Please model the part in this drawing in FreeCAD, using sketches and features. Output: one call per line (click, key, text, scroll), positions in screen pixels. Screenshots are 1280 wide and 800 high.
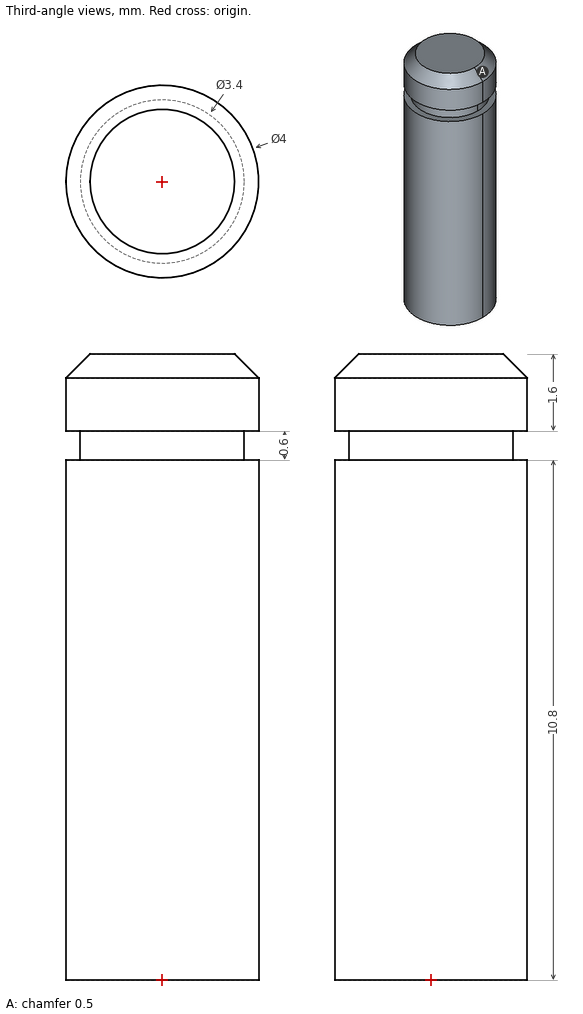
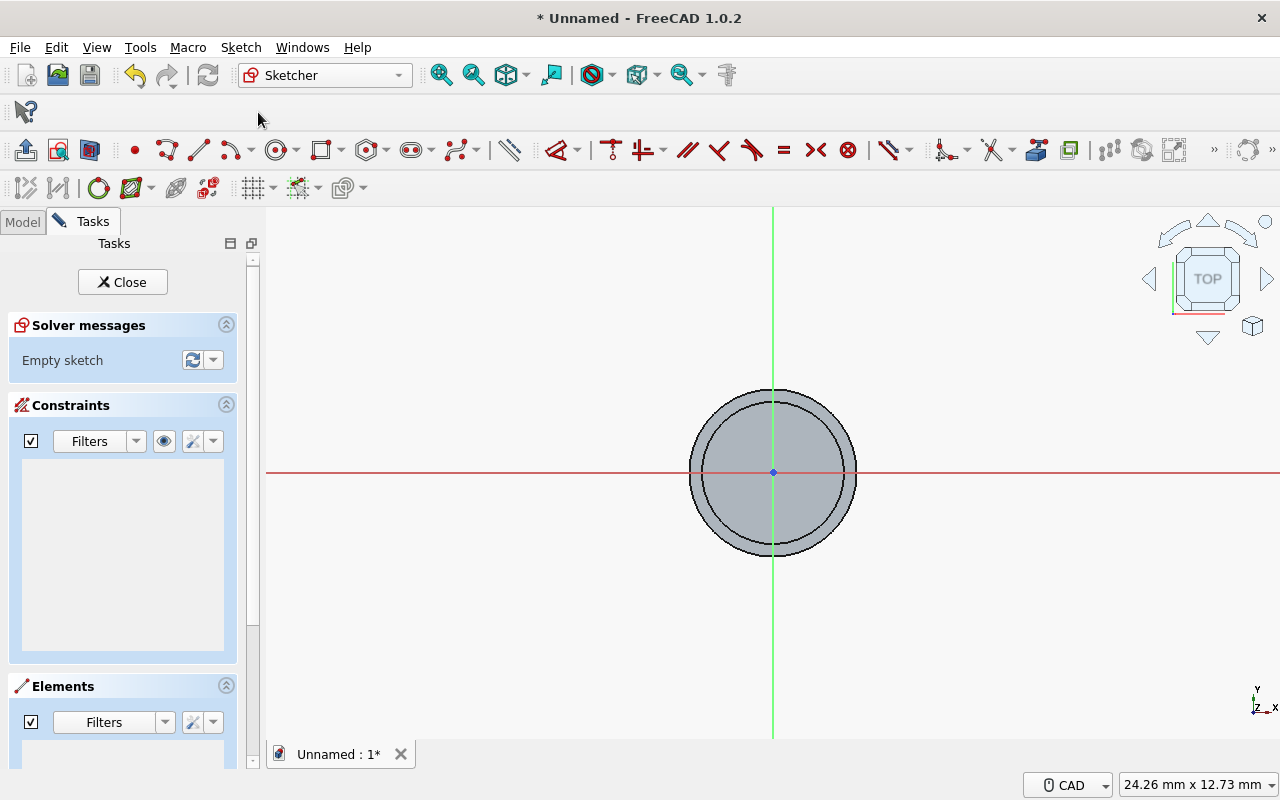
scroll(856, 473, up, 3)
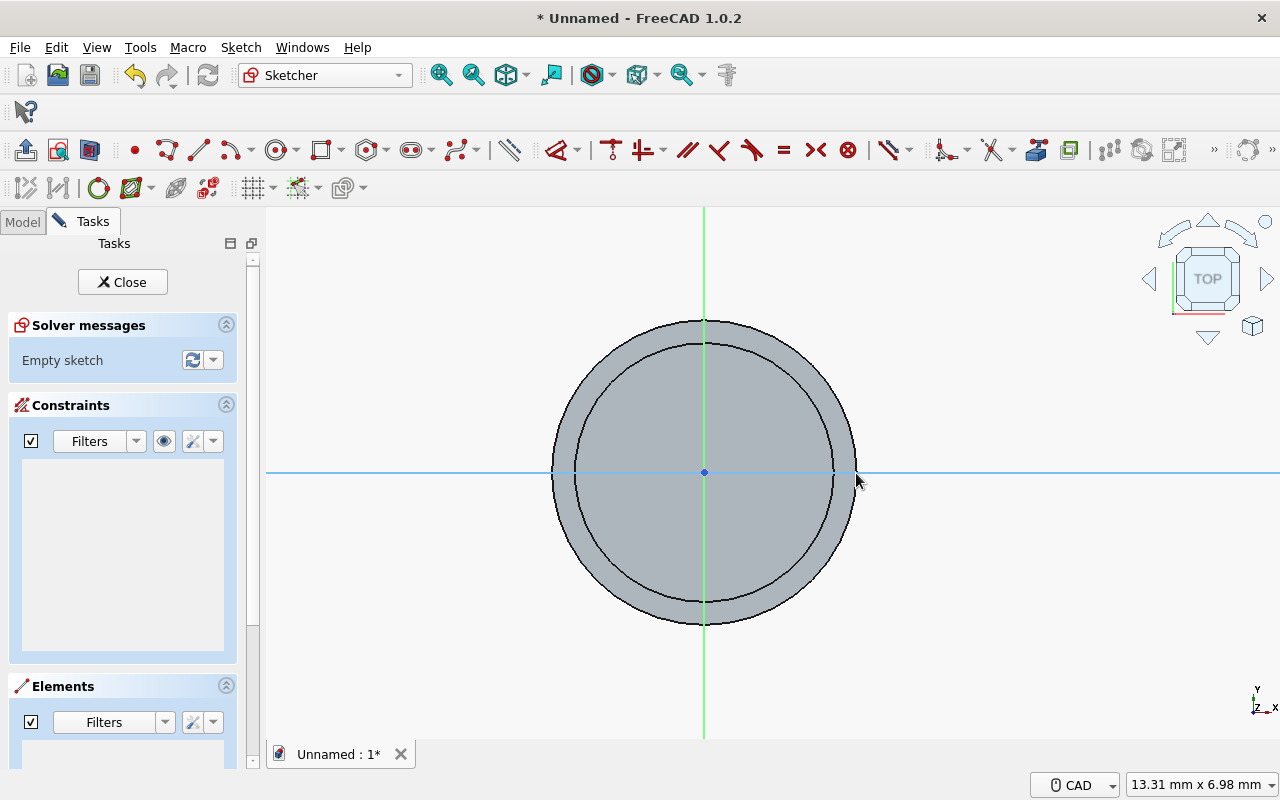
key(g)
key(c)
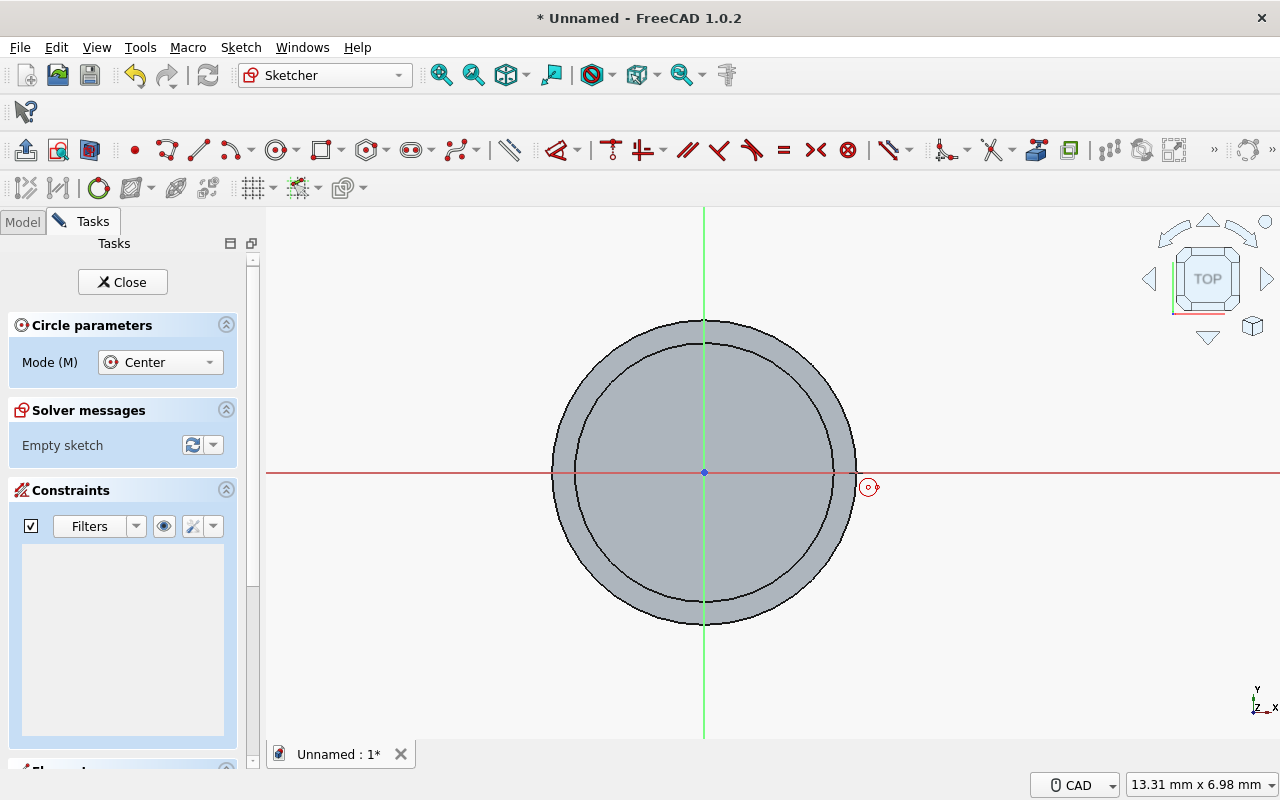
click(704, 473)
click(812, 365)
key(Escape)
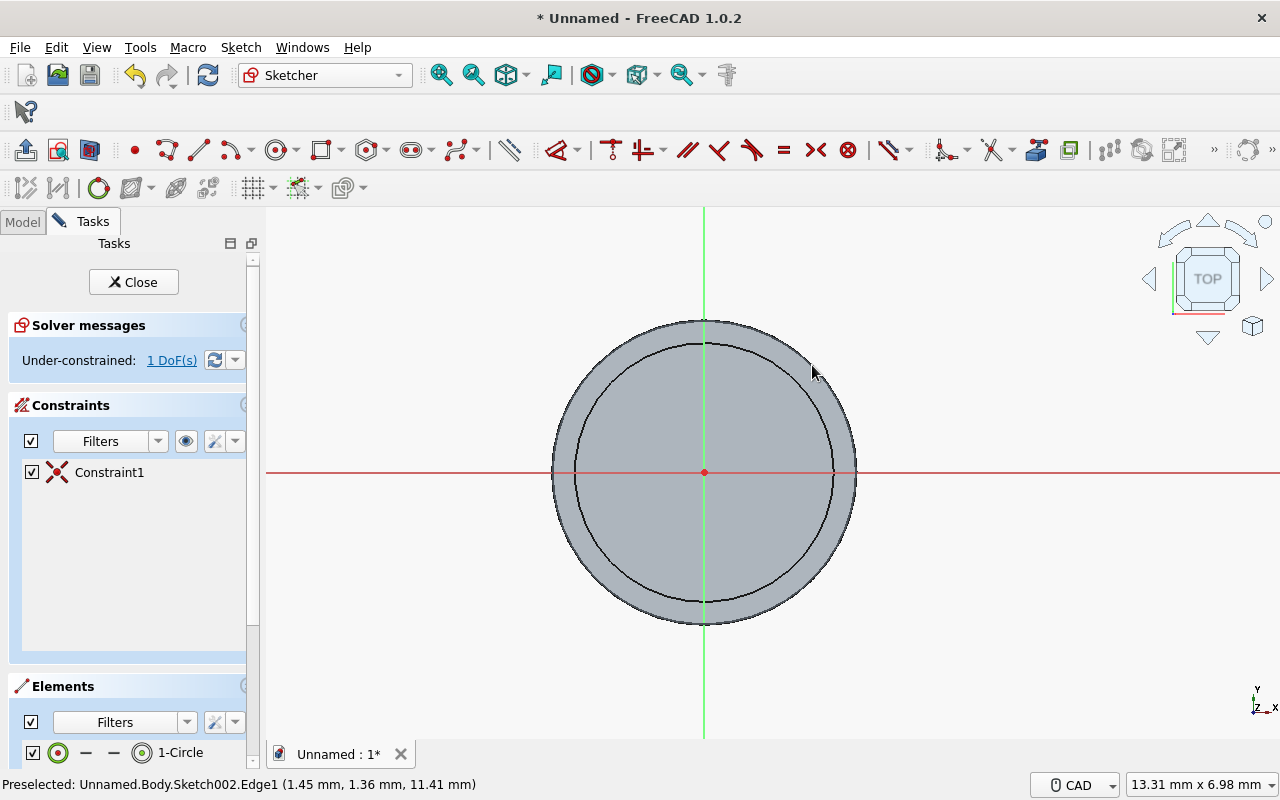
key(d)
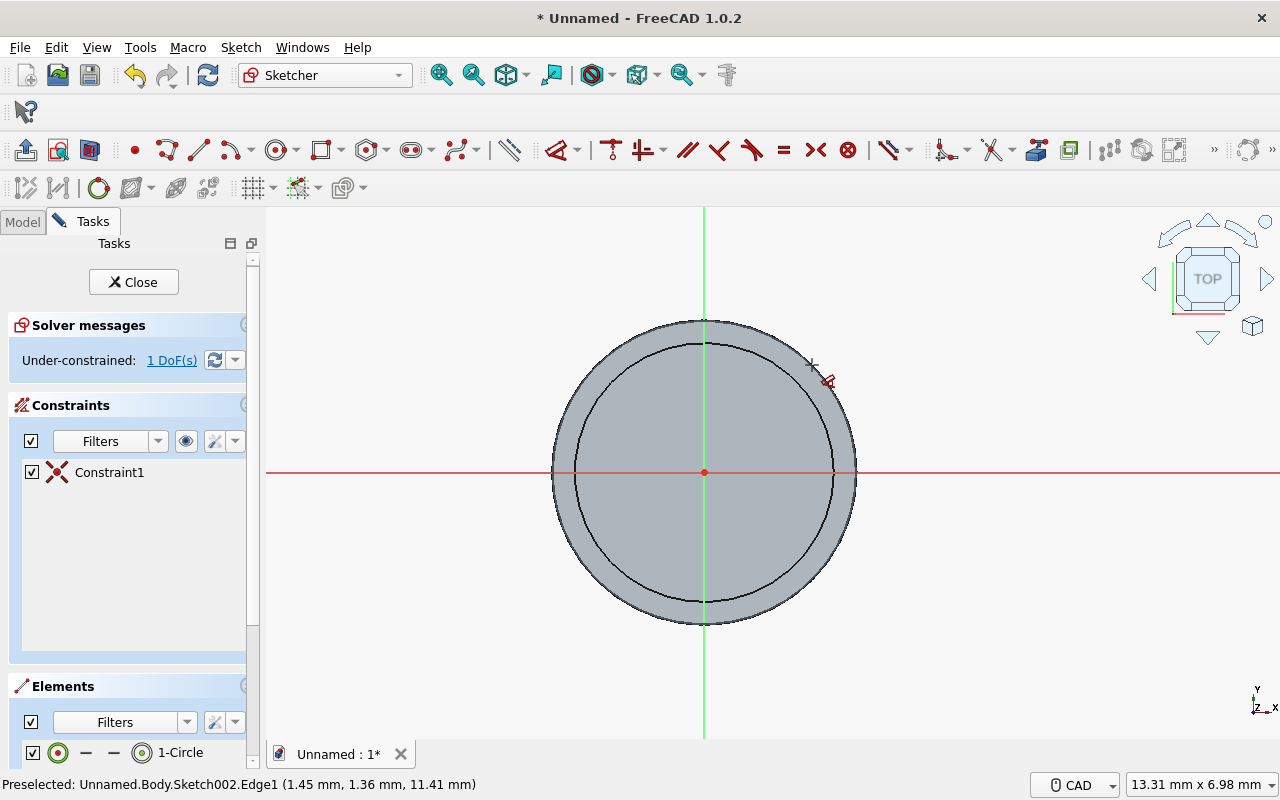
click(811, 365)
click(834, 342)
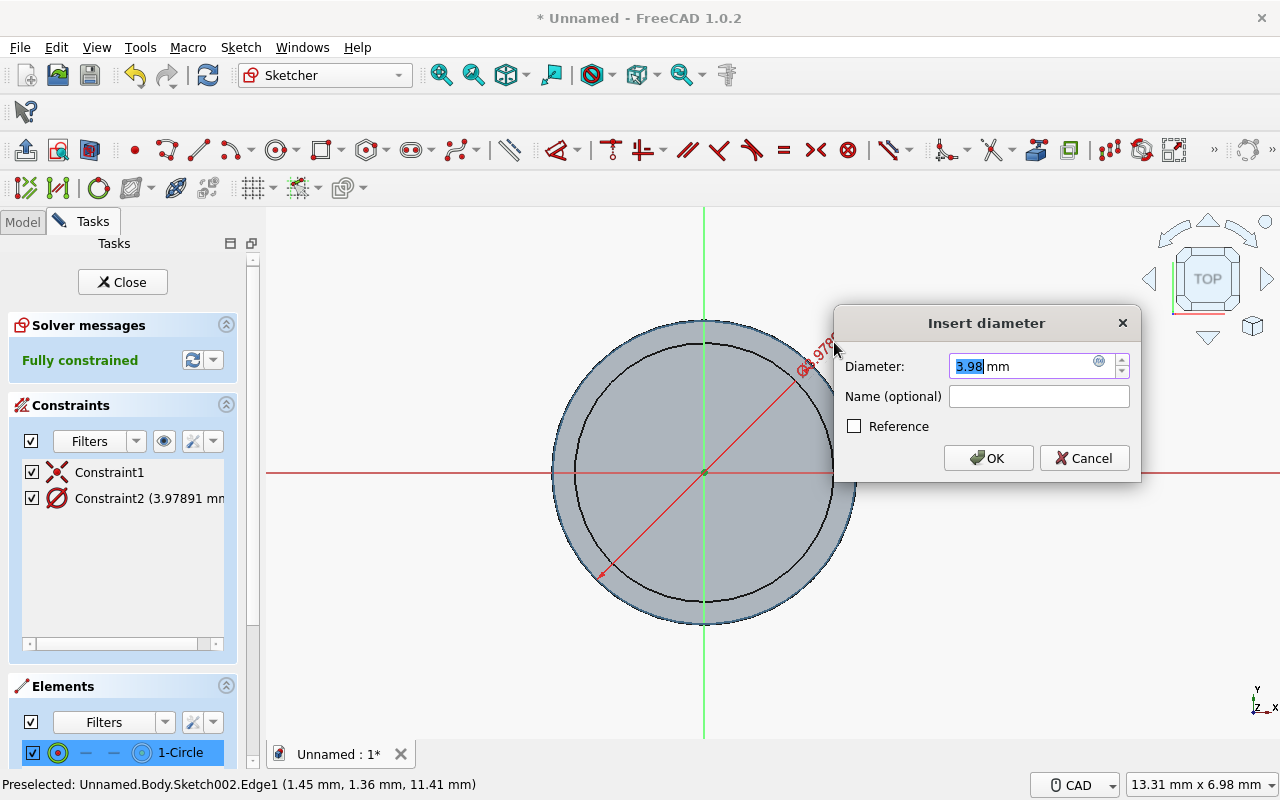
text(4)
key(Return)
key(Escape)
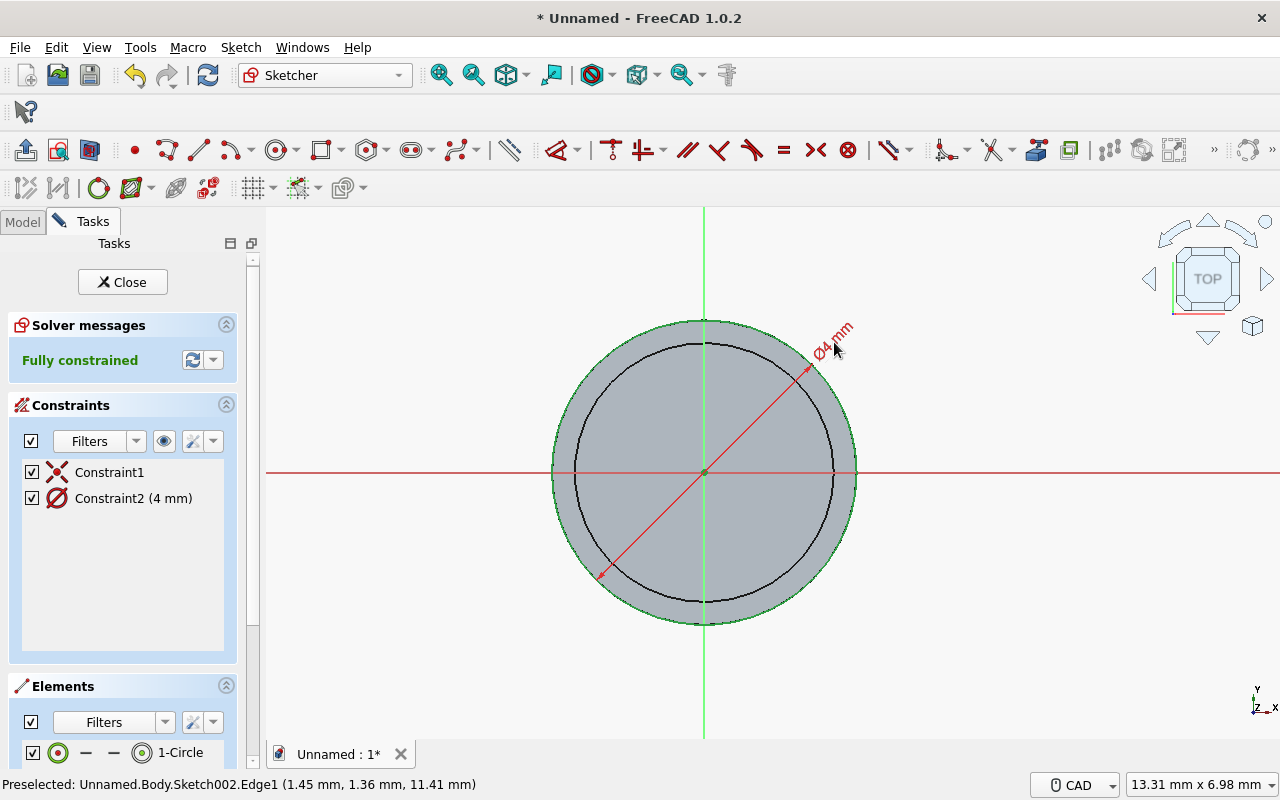
click(123, 282)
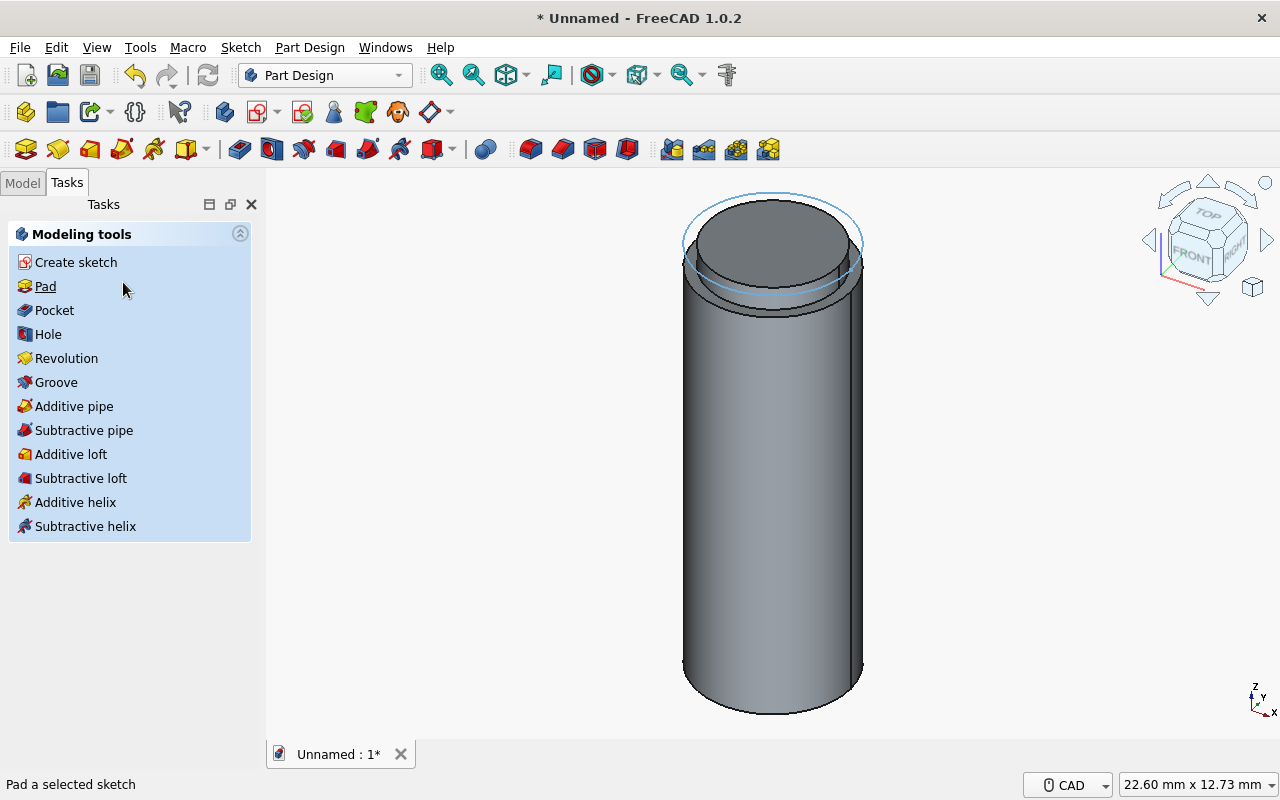
click(26, 150)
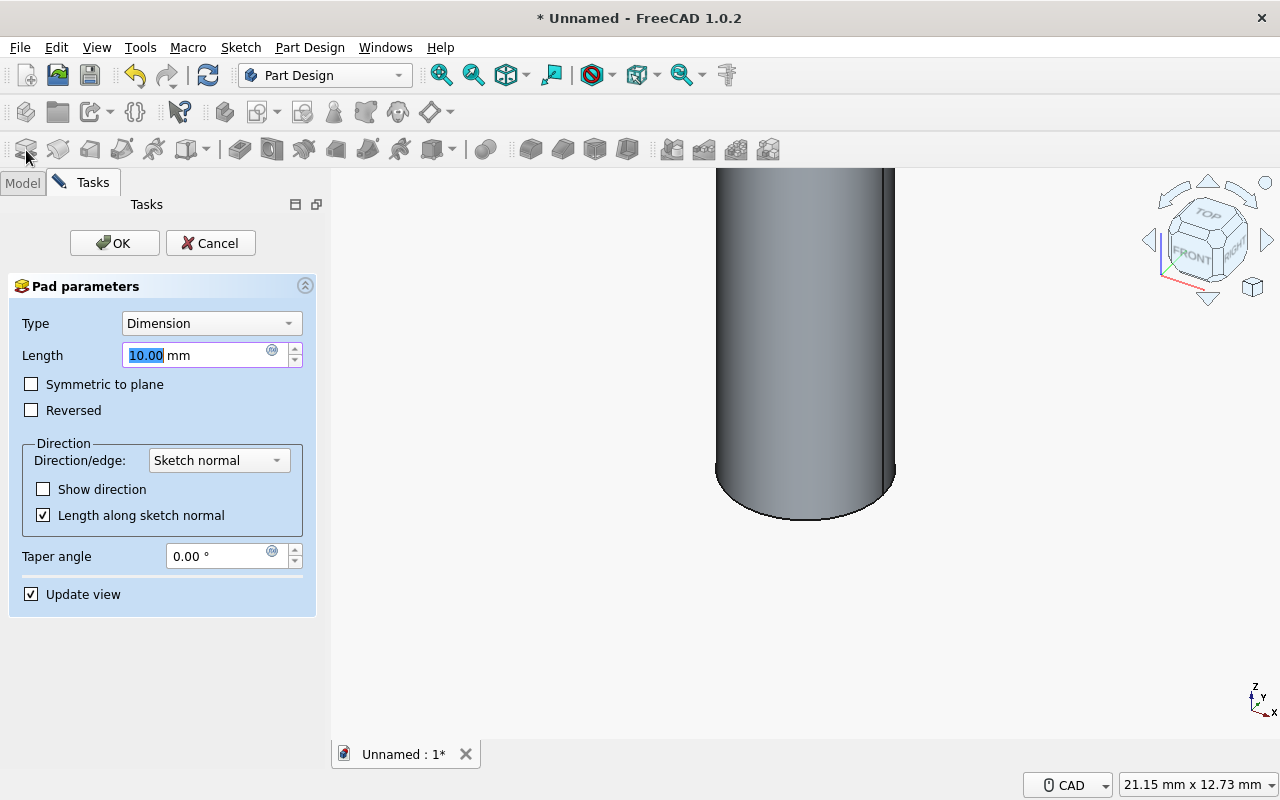
text(1.6)
key(Tab)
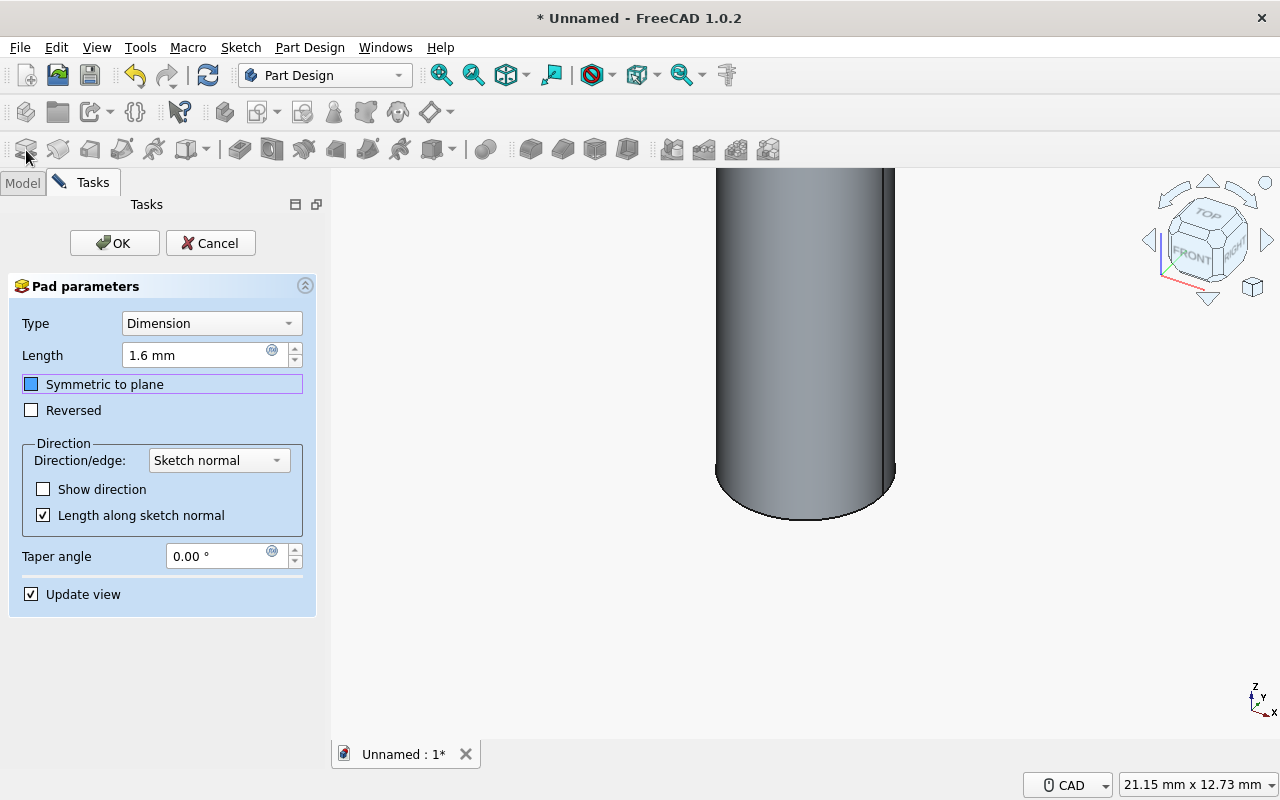
click(115, 243)